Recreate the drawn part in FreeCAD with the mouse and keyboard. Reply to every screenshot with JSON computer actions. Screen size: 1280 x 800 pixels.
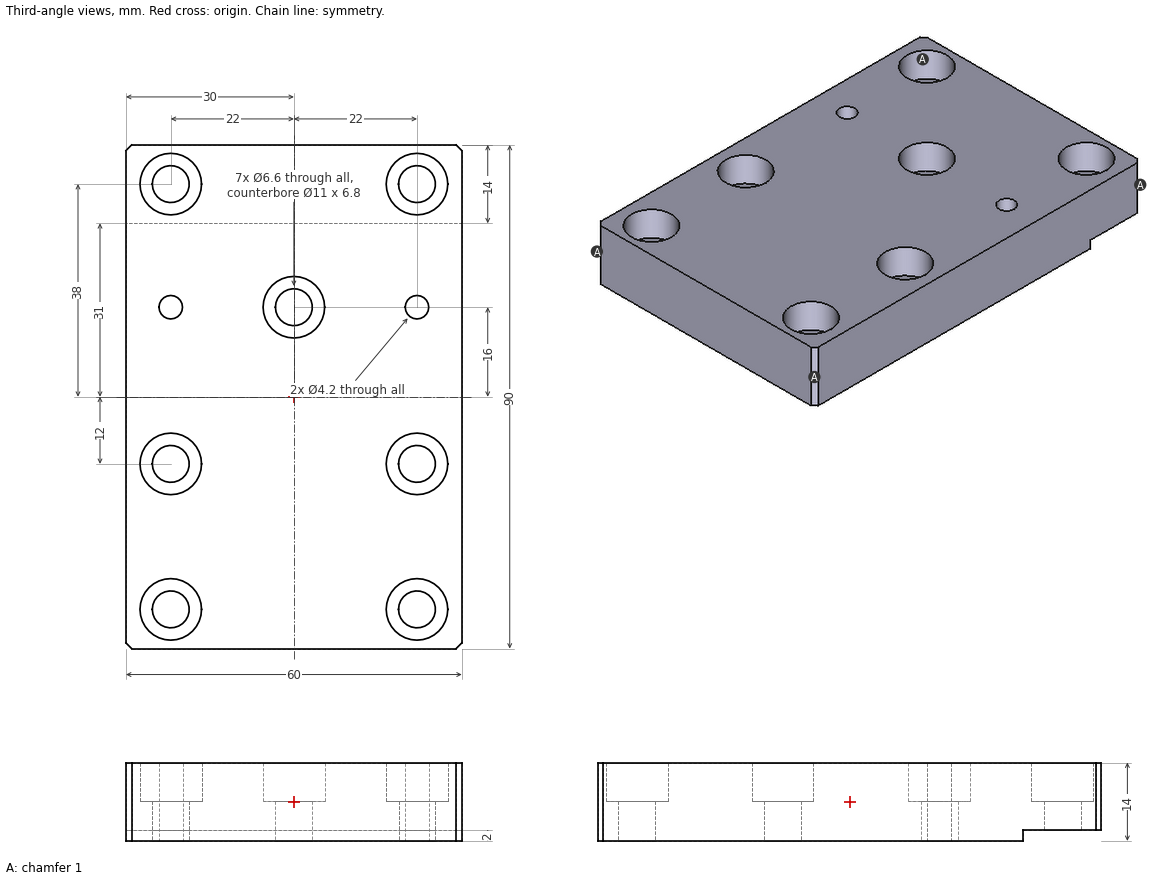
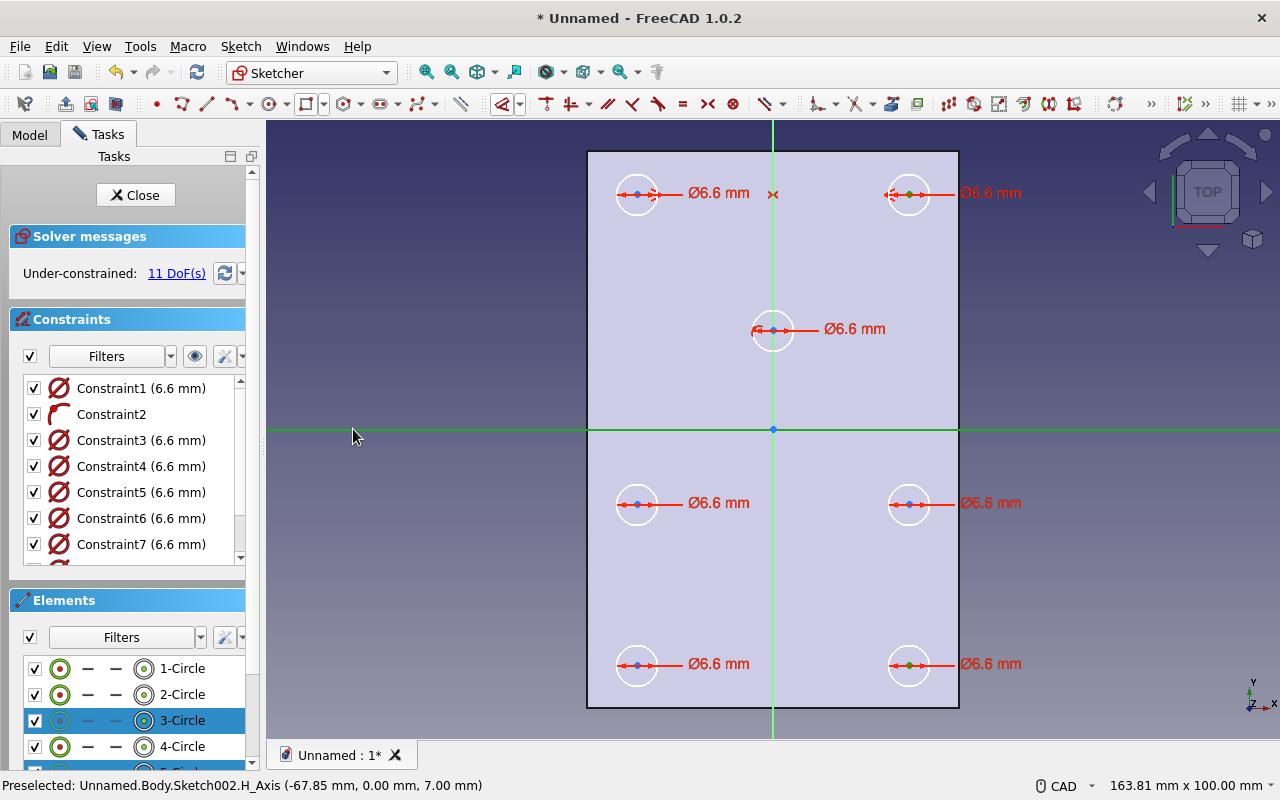
{"action": "left_click", "coordinate": [708, 104]}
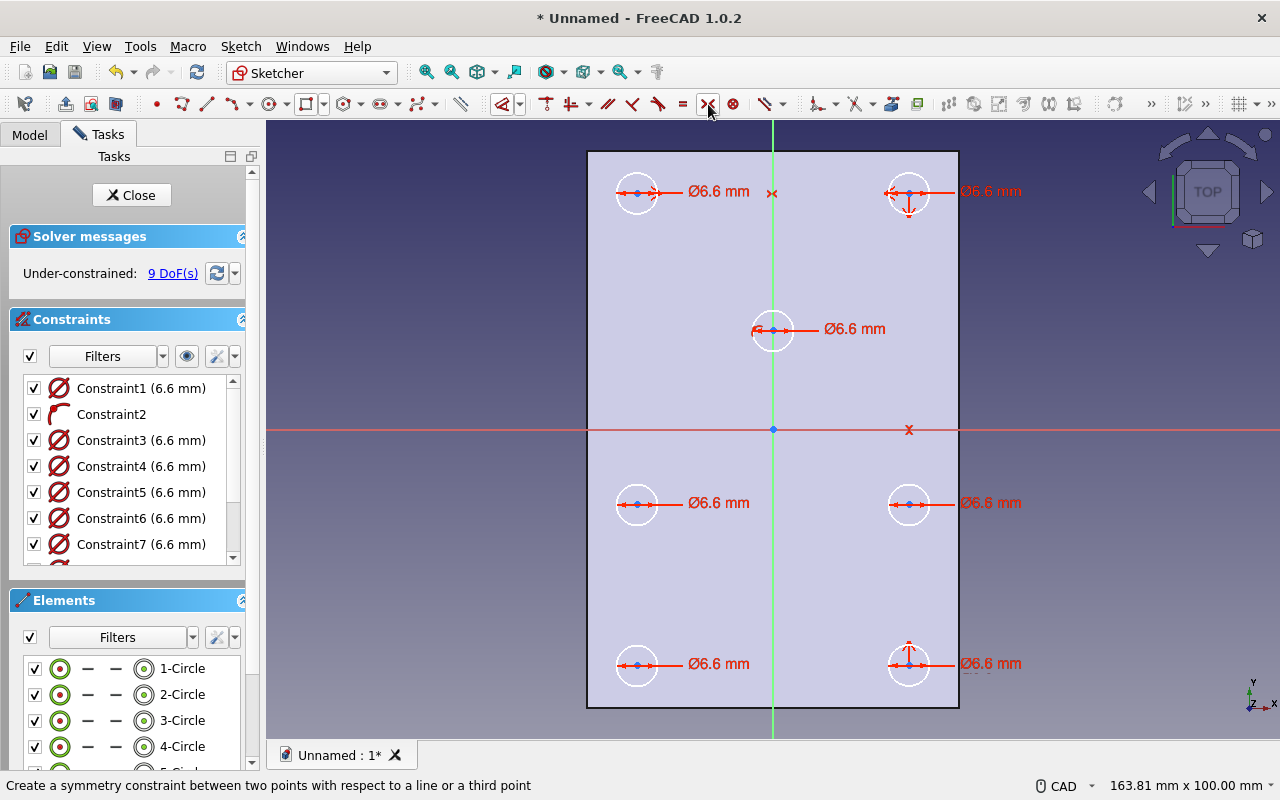
{"action": "left_click", "coordinate": [637, 193]}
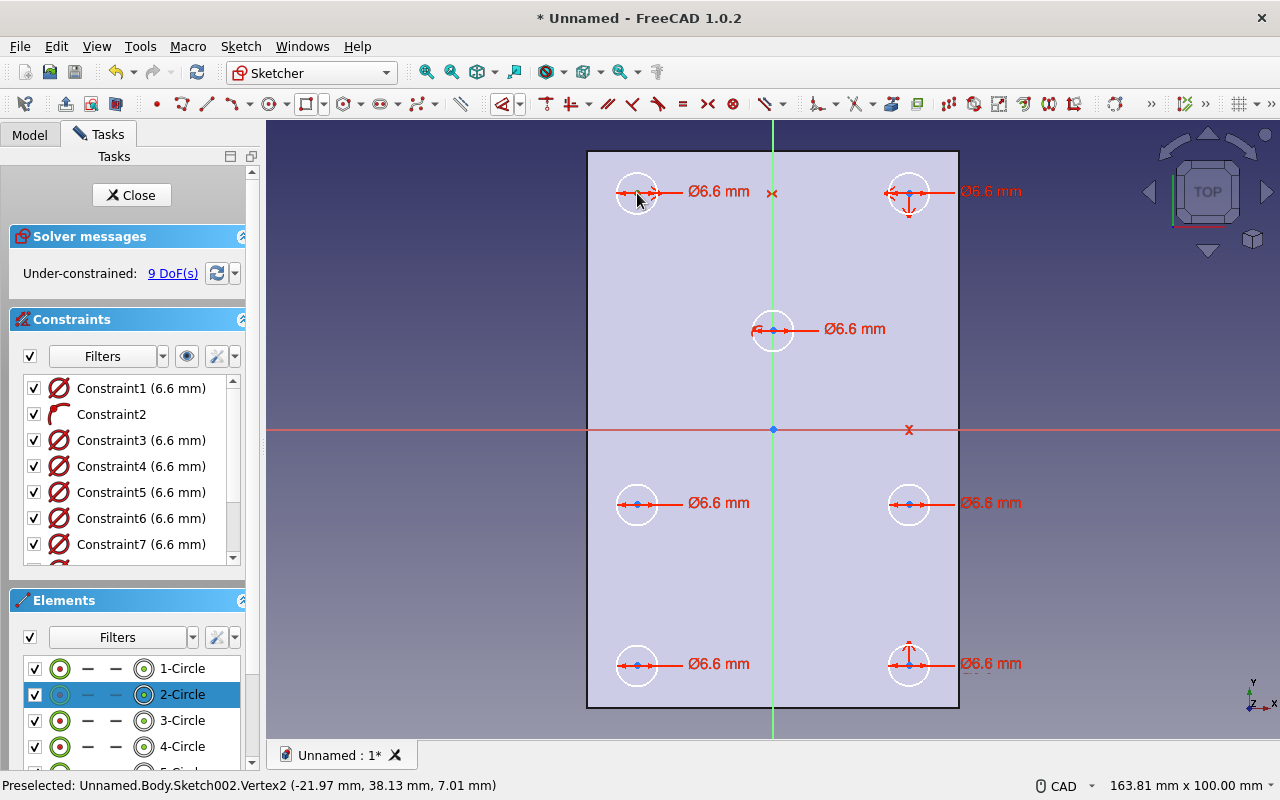
{"action": "left_click", "coordinate": [637, 666]}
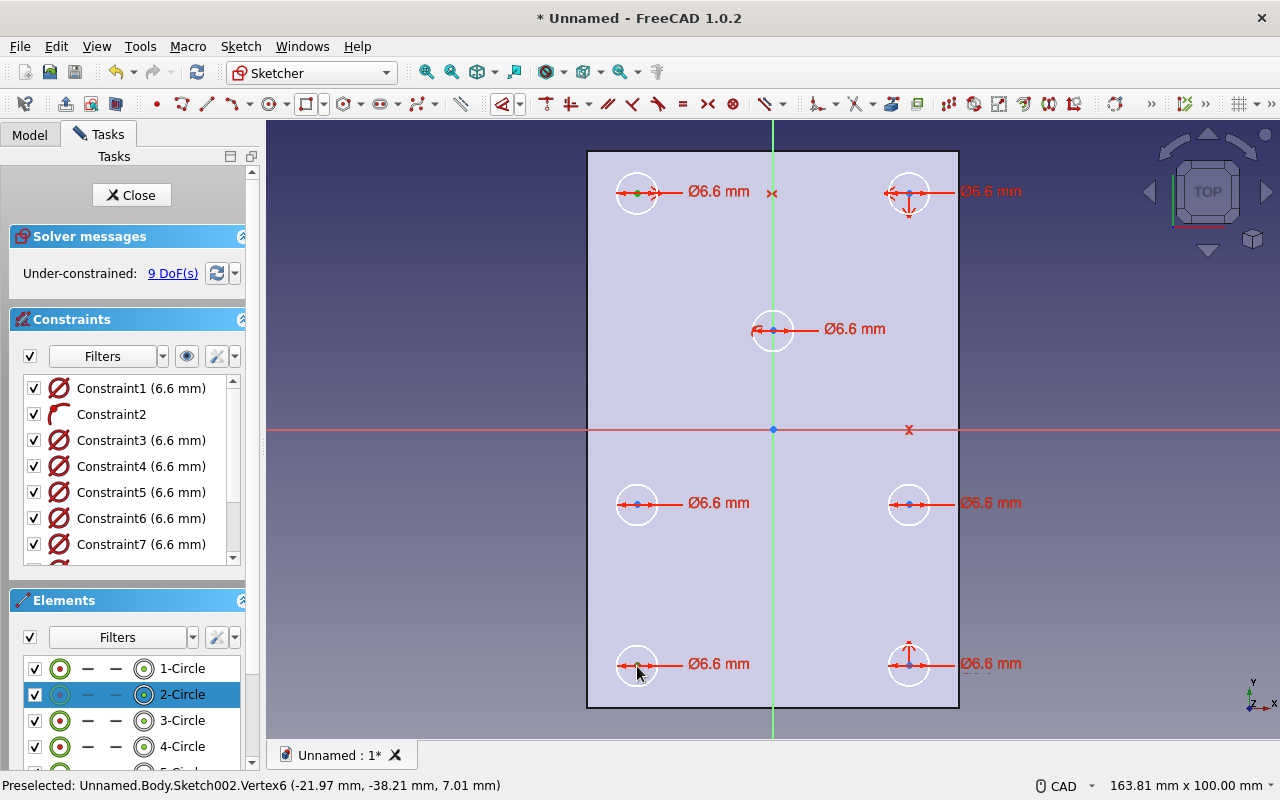
{"action": "left_click", "coordinate": [353, 429]}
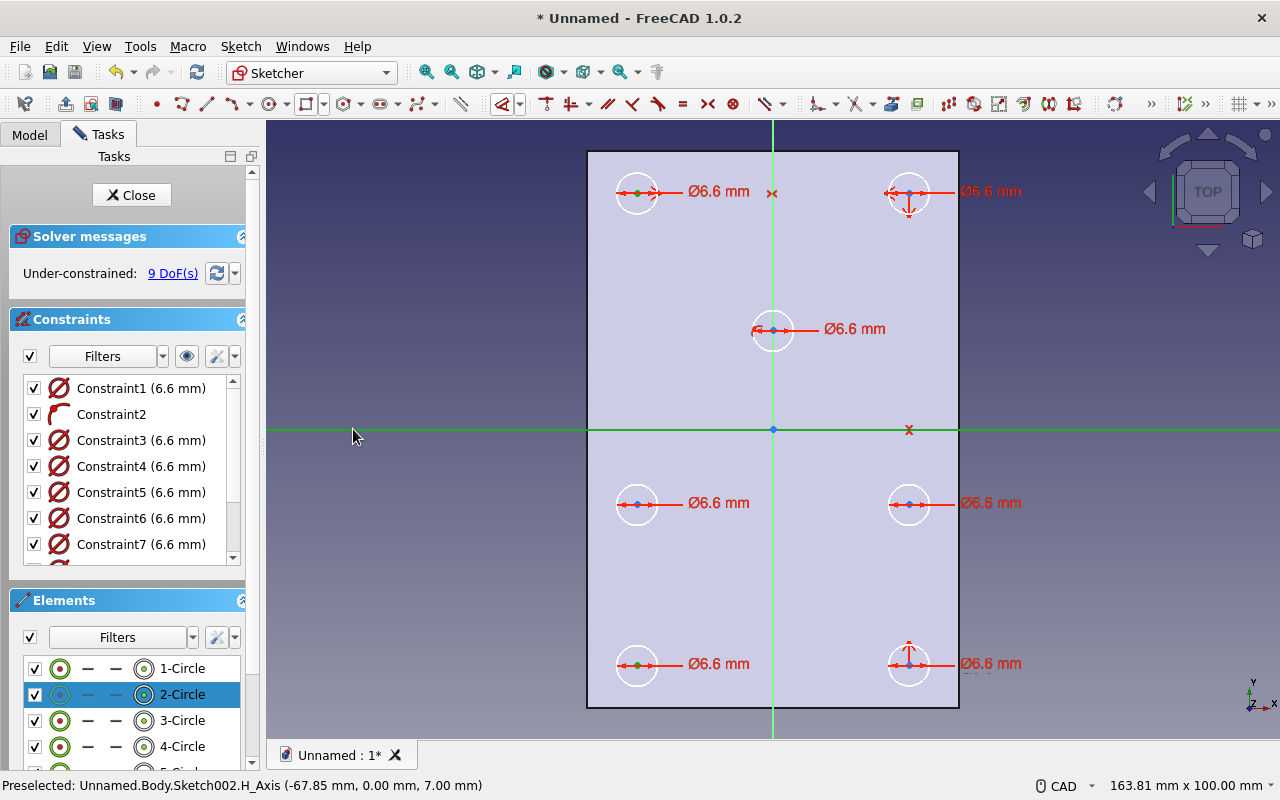
{"action": "left_click", "coordinate": [708, 104]}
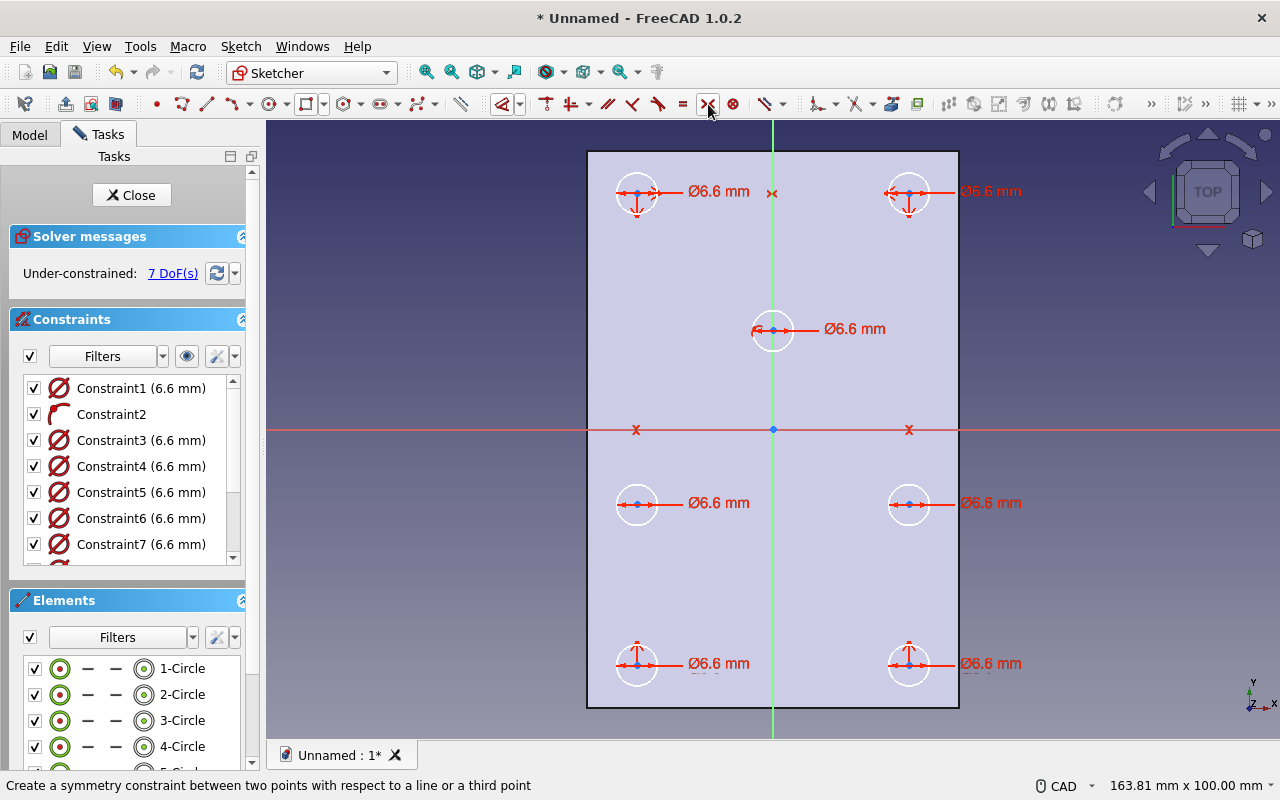
{"action": "left_click", "coordinate": [637, 505]}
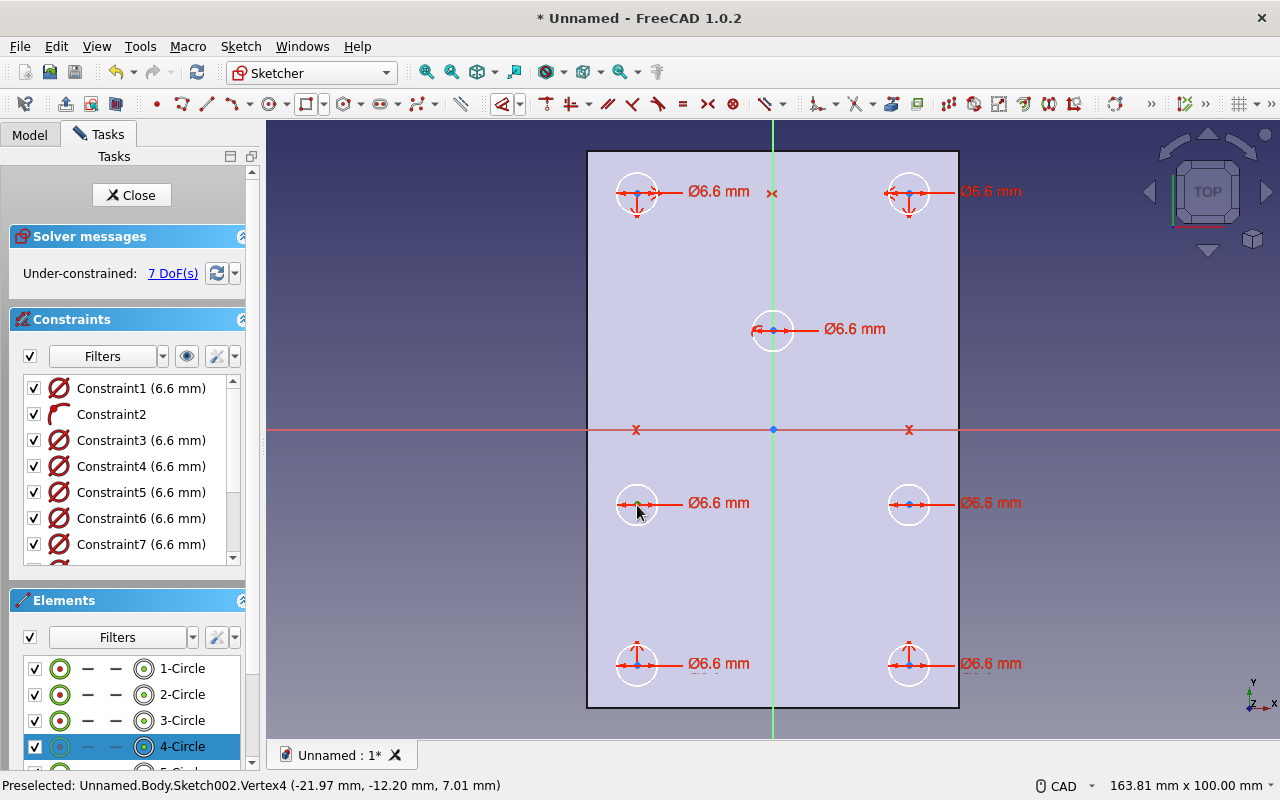
{"action": "left_click", "coordinate": [909, 505]}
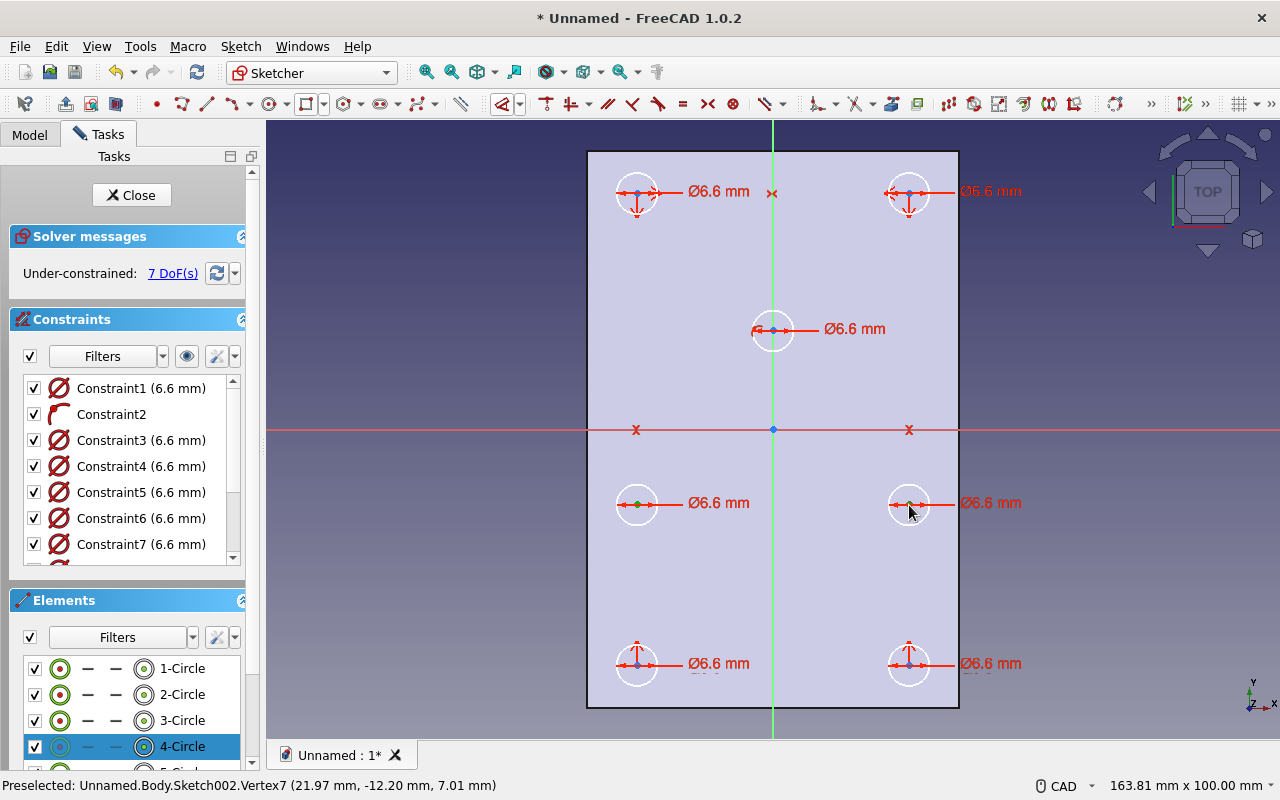
{"action": "left_click", "coordinate": [773, 671]}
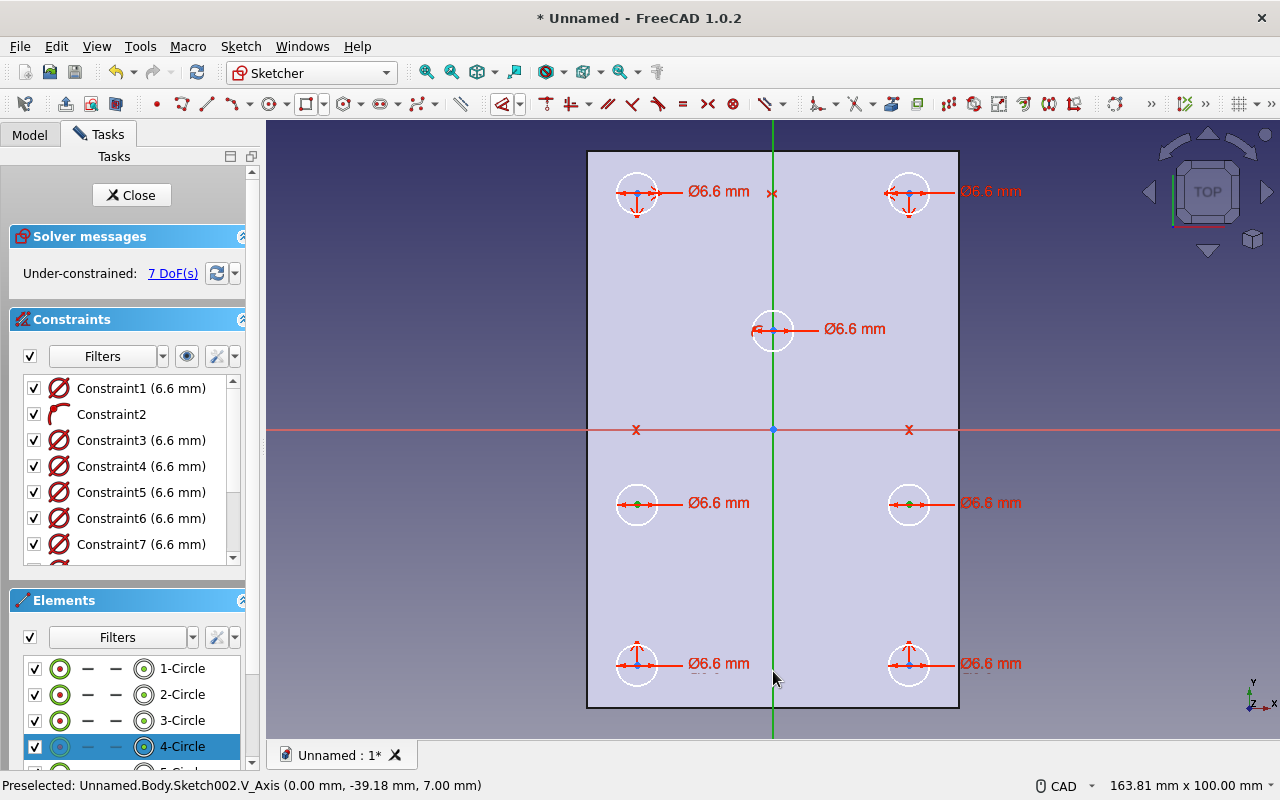
{"action": "left_click", "coordinate": [708, 104]}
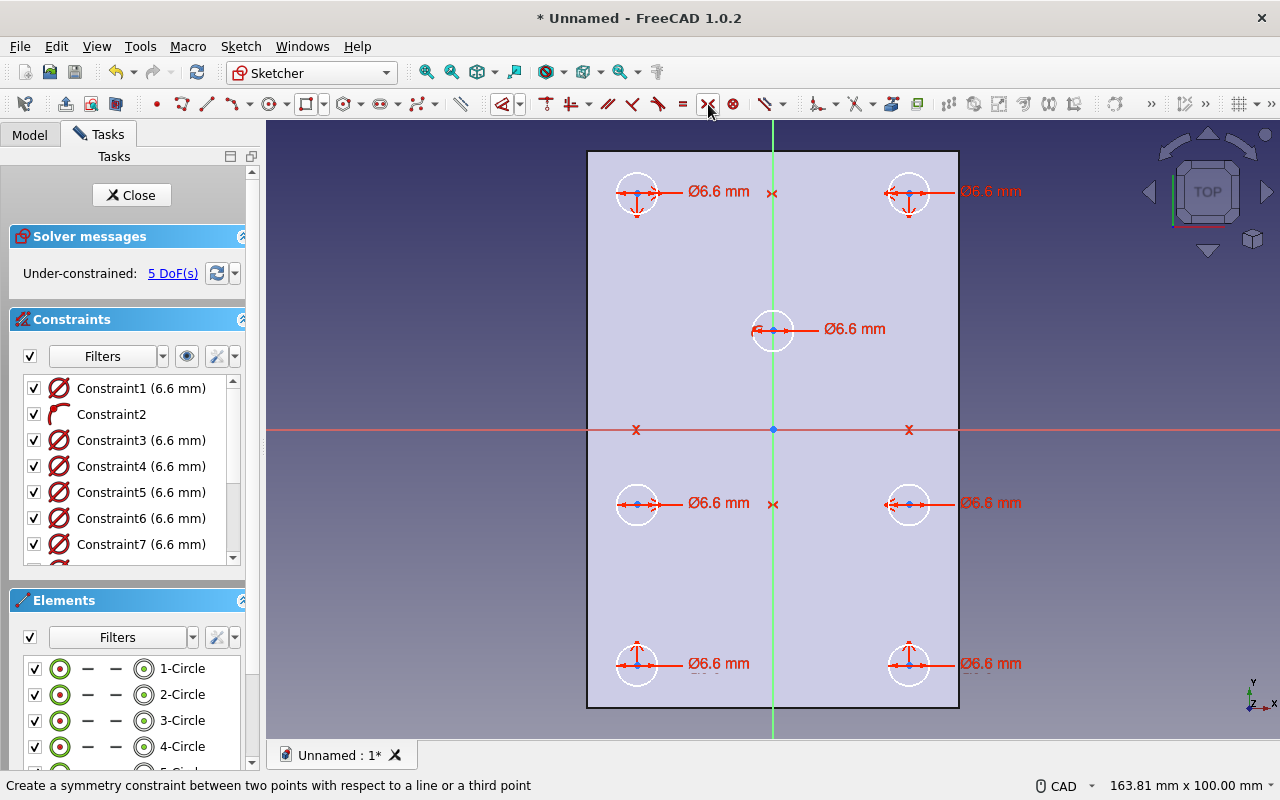
{"action": "left_click", "coordinate": [773, 331]}